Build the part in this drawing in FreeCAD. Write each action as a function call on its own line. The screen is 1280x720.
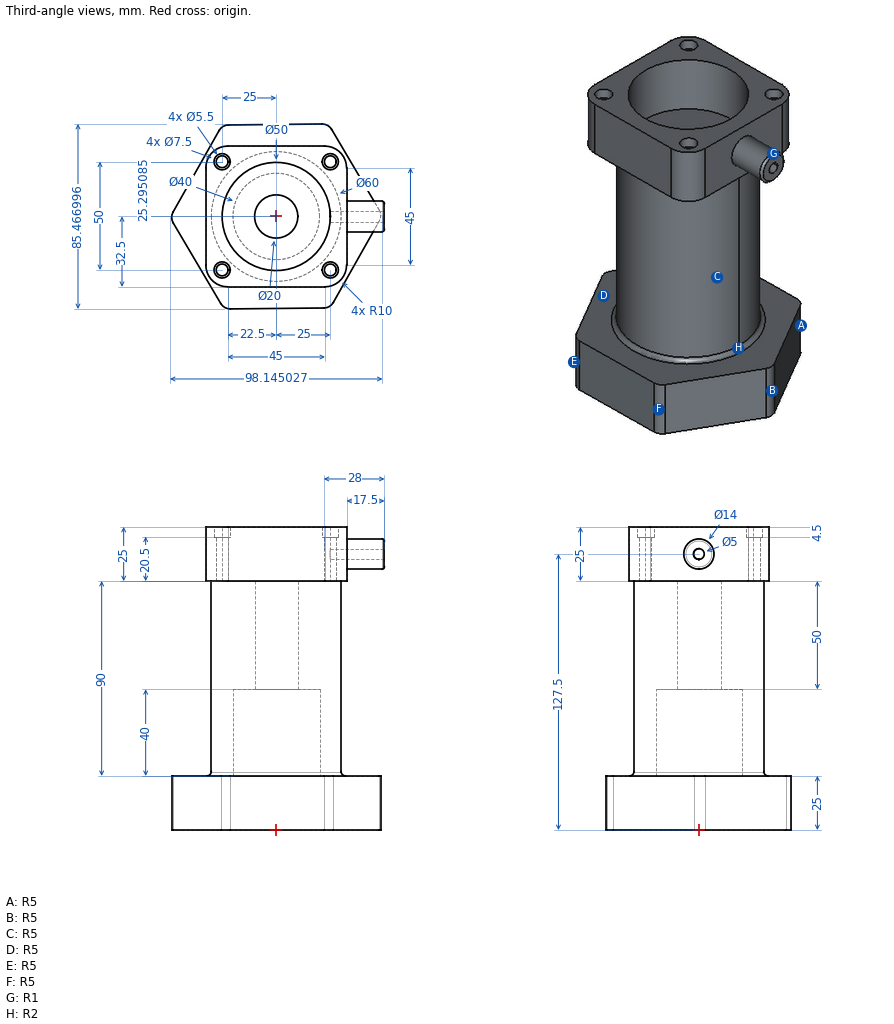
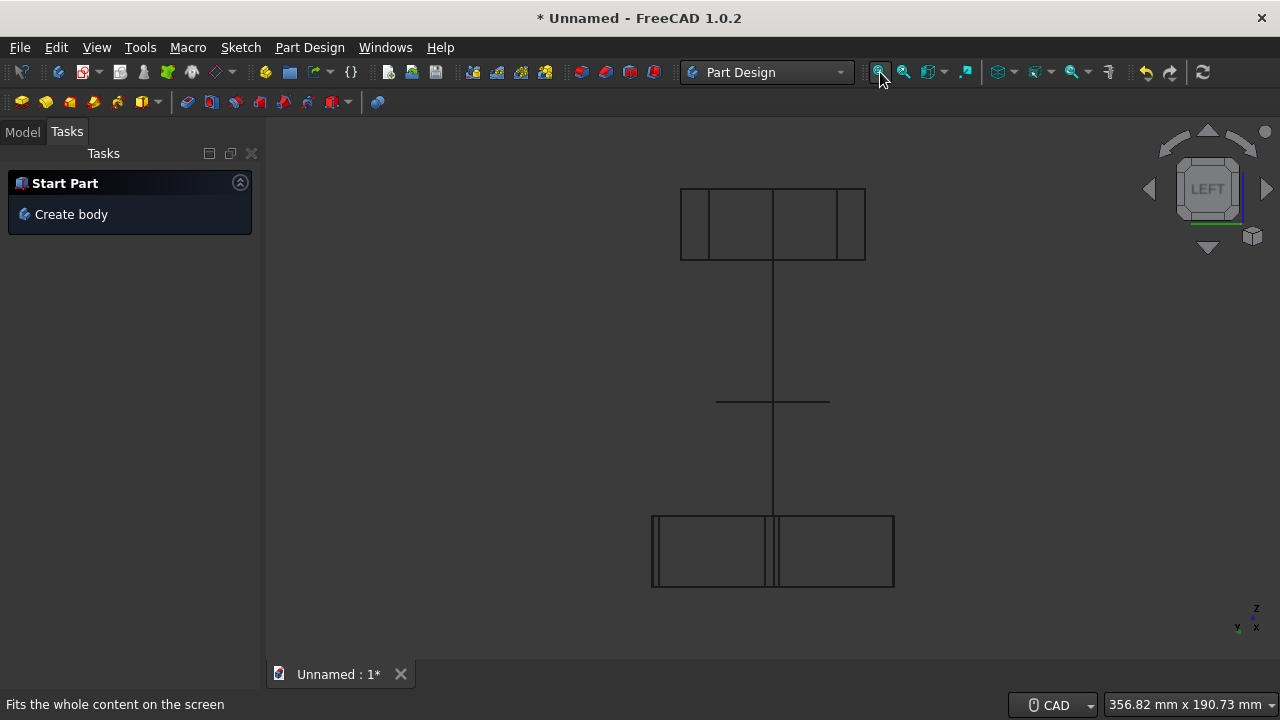
key(0)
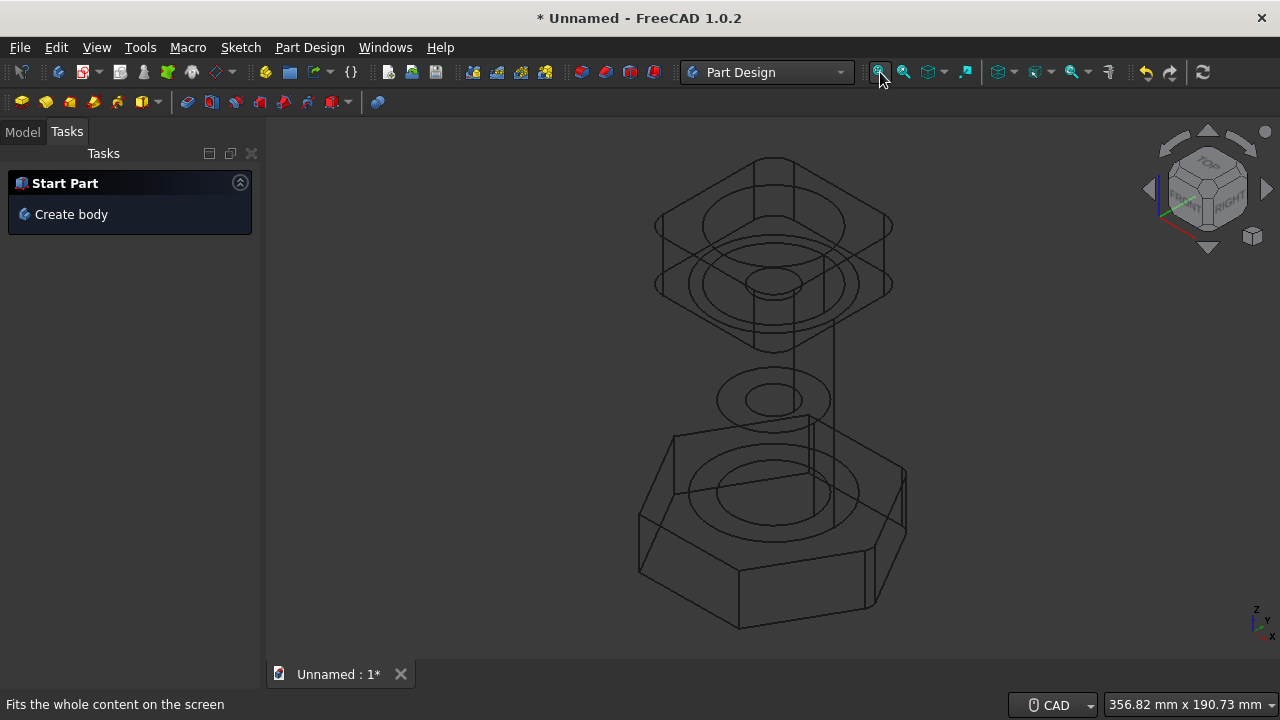
scroll(809, 443, up, 6)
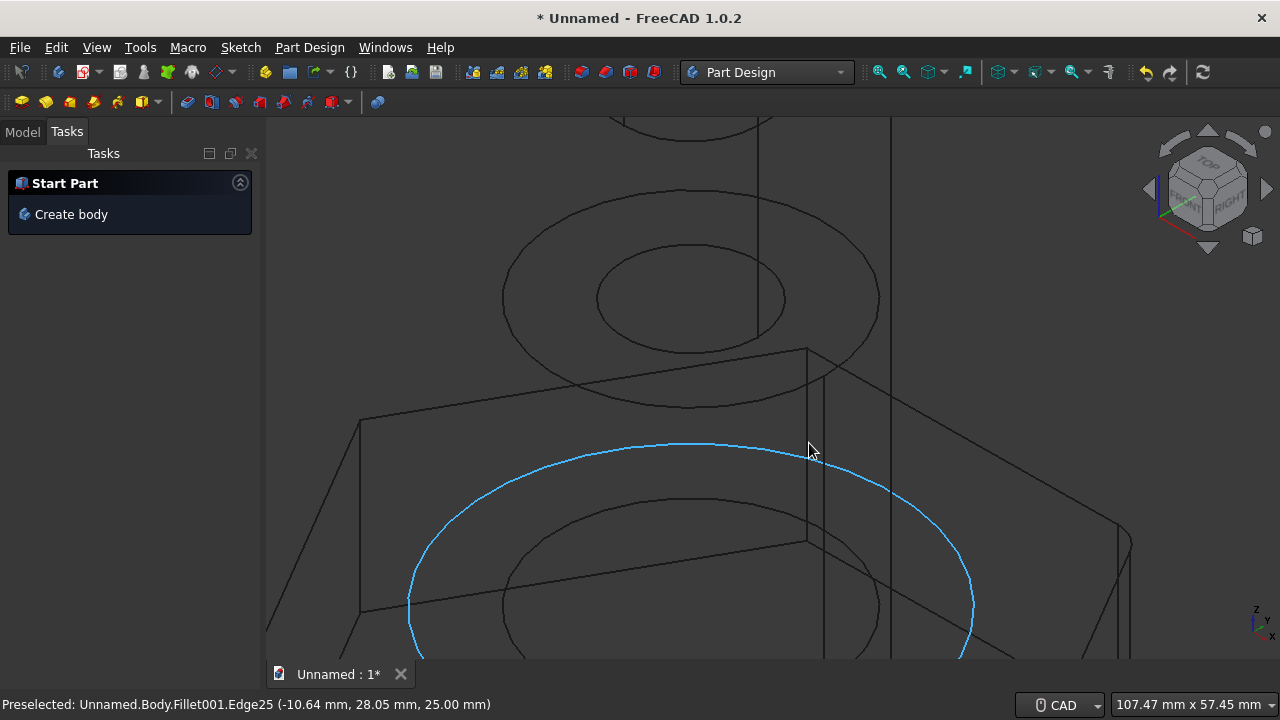
click(807, 444)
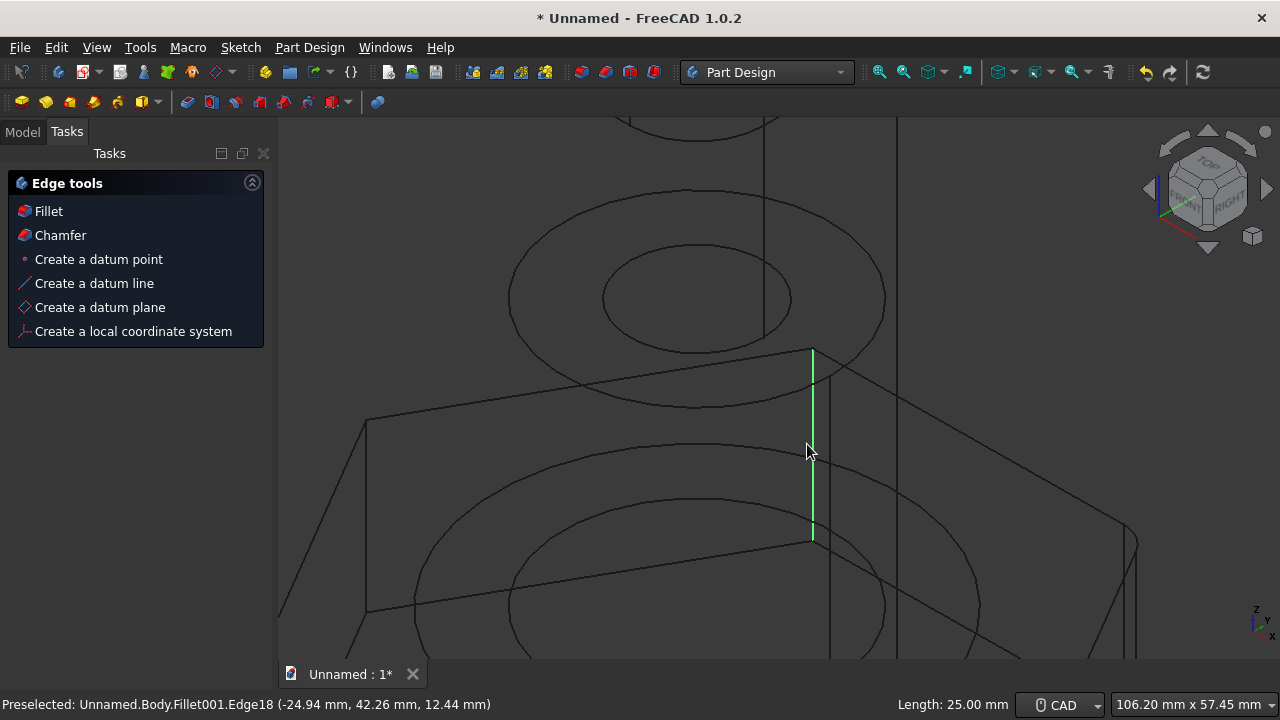
key(v)
key(1)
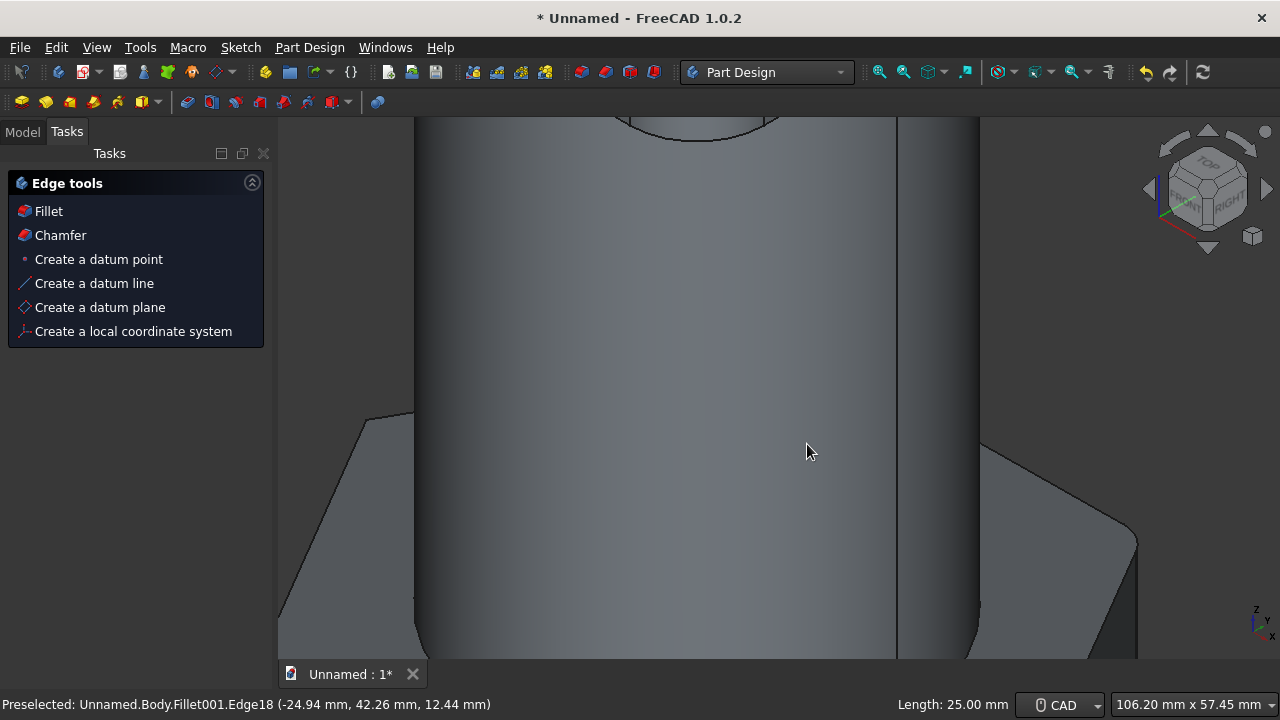
click(582, 72)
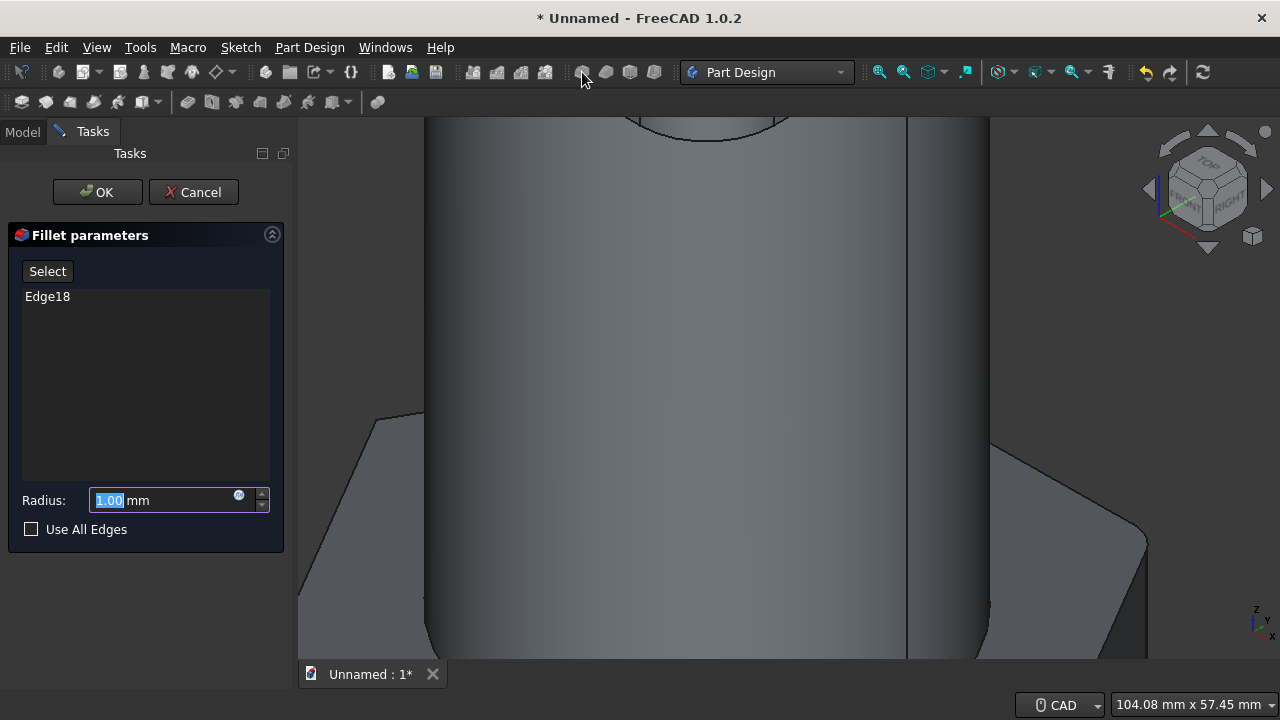
text(5)
key(Tab)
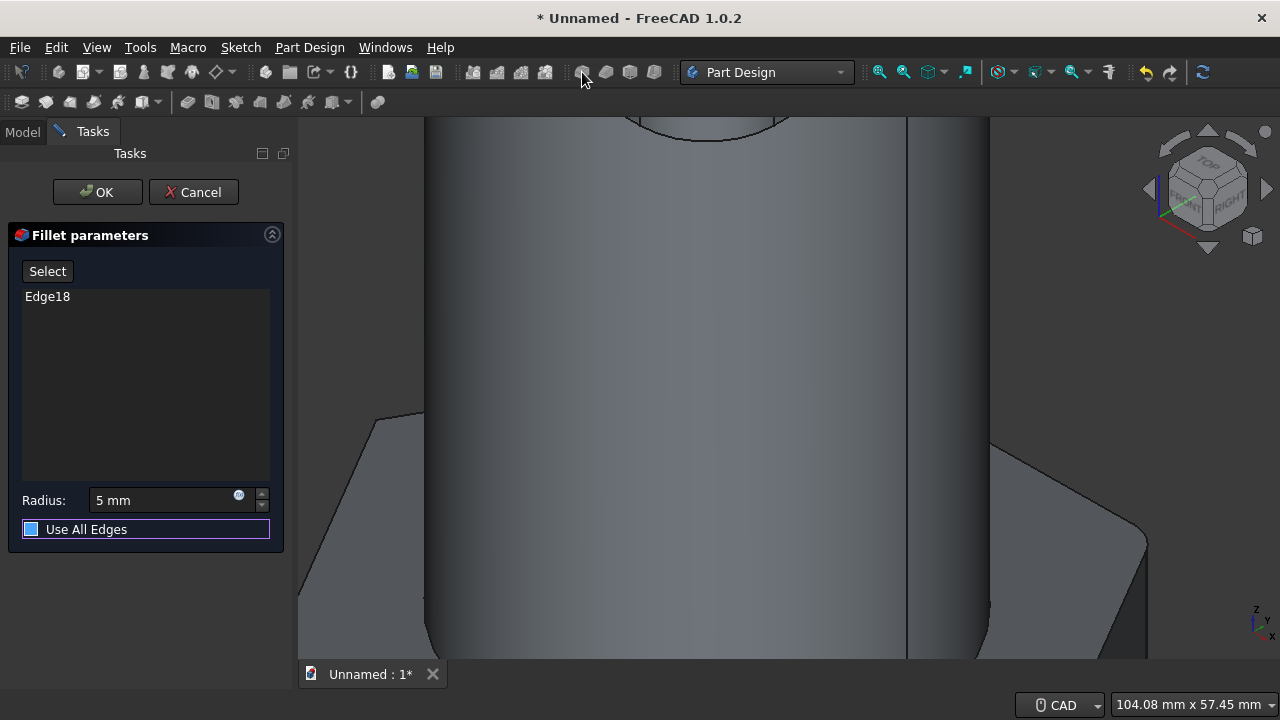
click(98, 192)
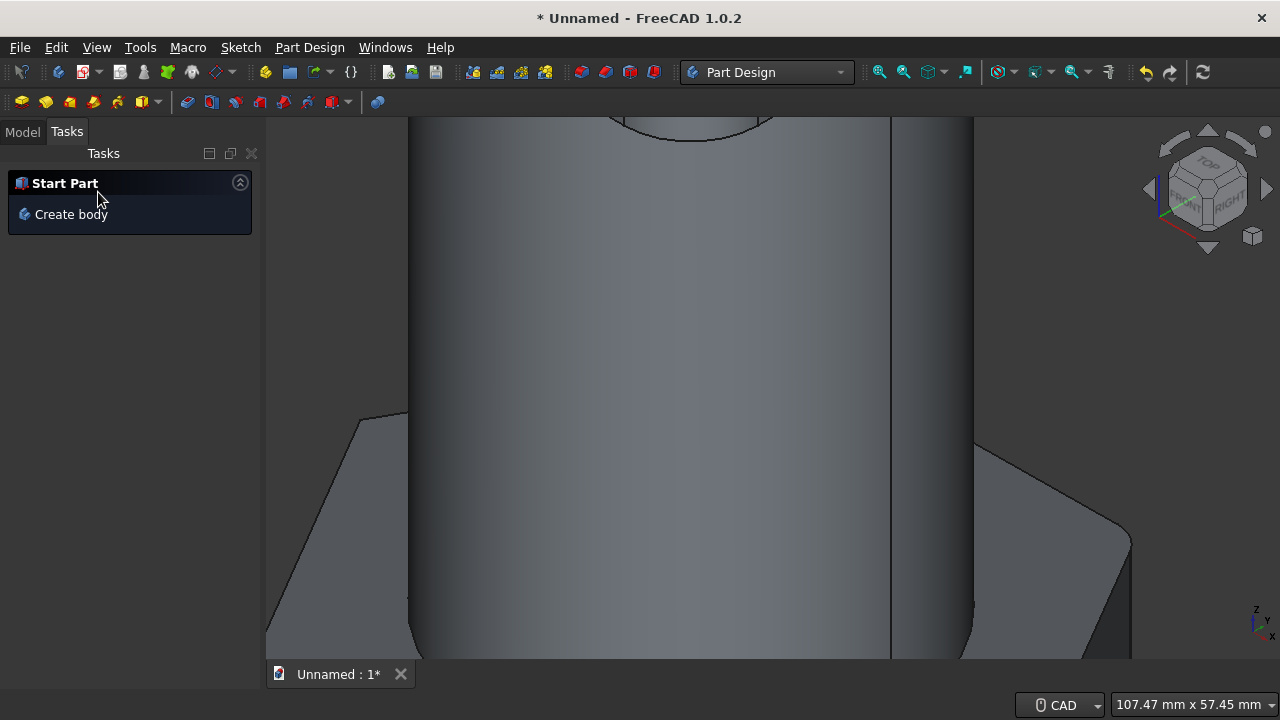
click(880, 72)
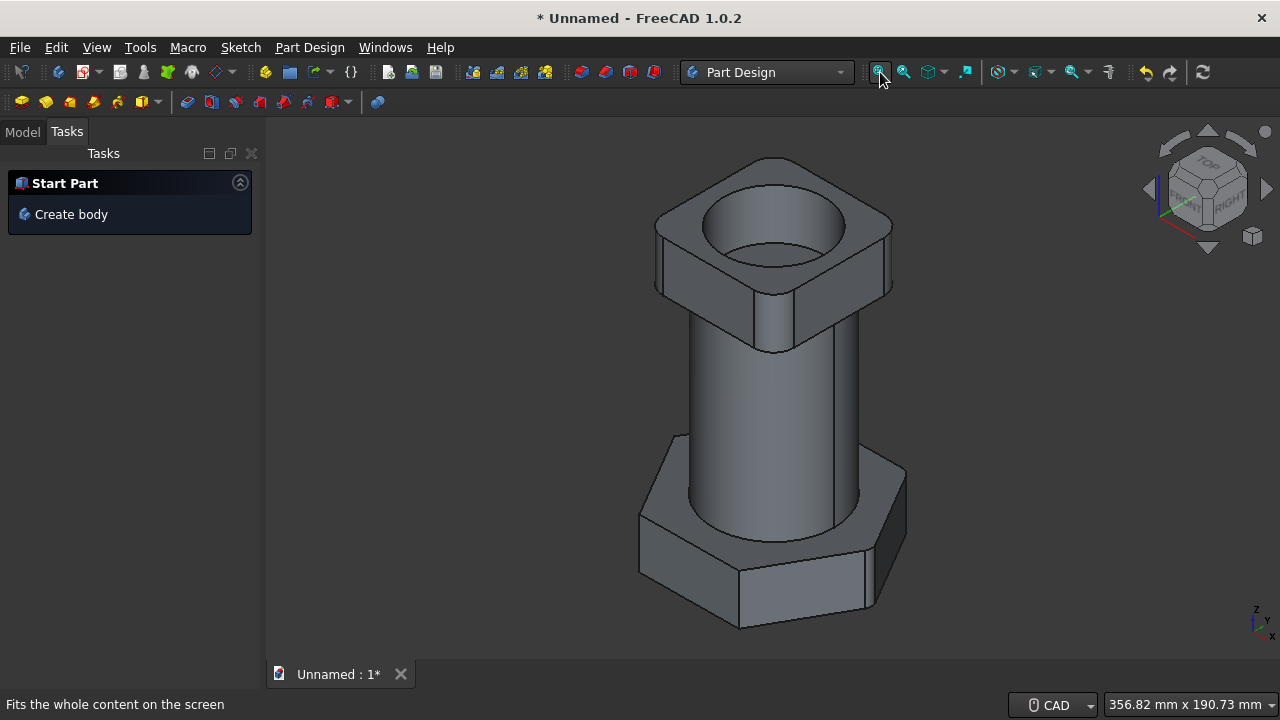
key(2)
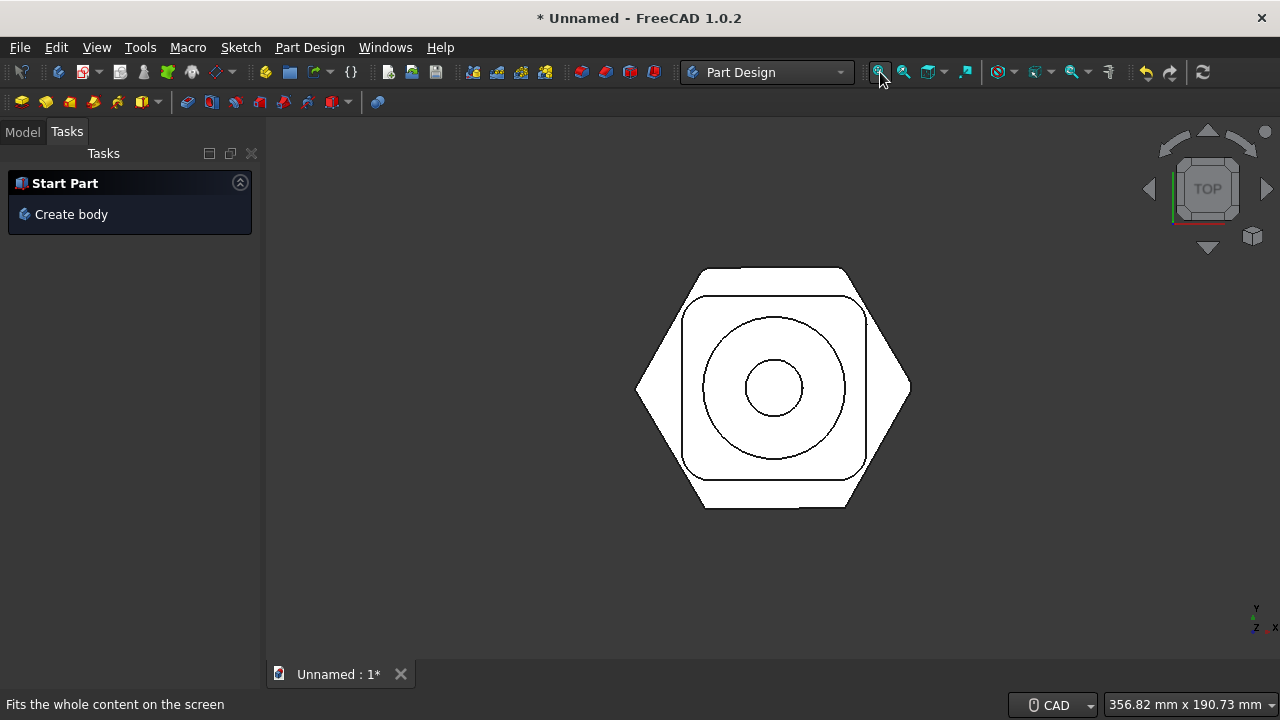
key(v)
key(f)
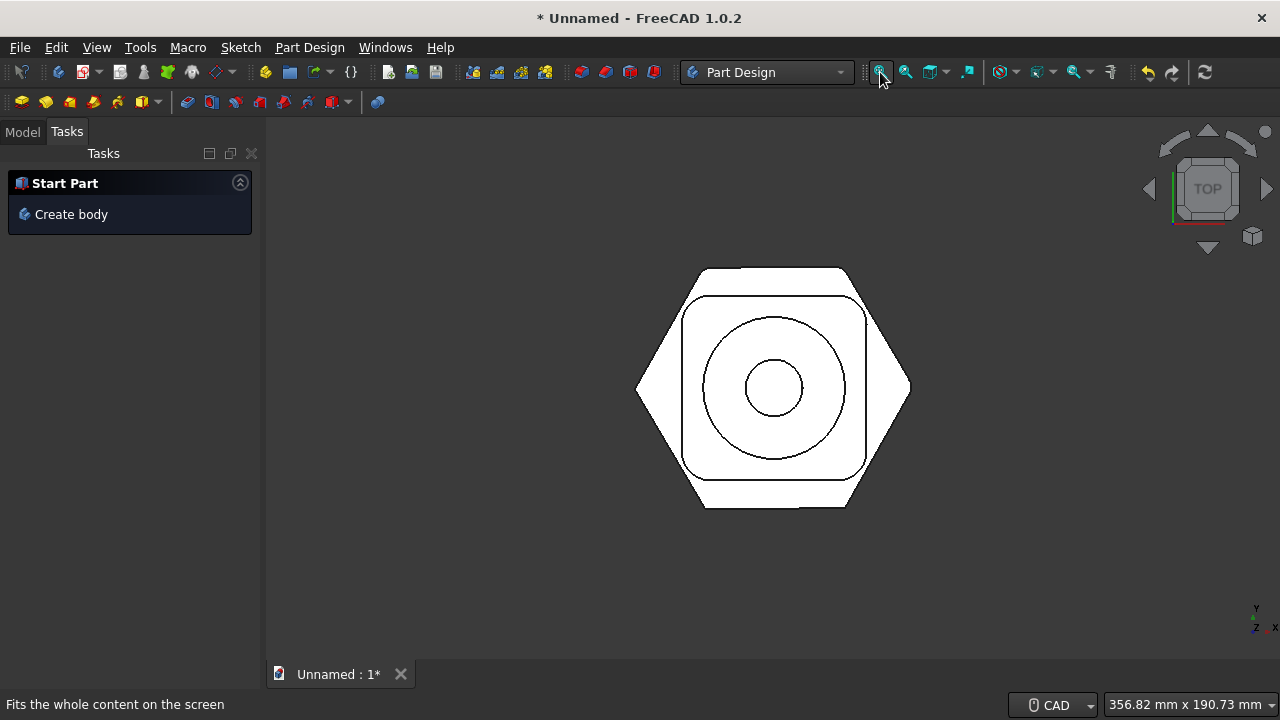
key(0)